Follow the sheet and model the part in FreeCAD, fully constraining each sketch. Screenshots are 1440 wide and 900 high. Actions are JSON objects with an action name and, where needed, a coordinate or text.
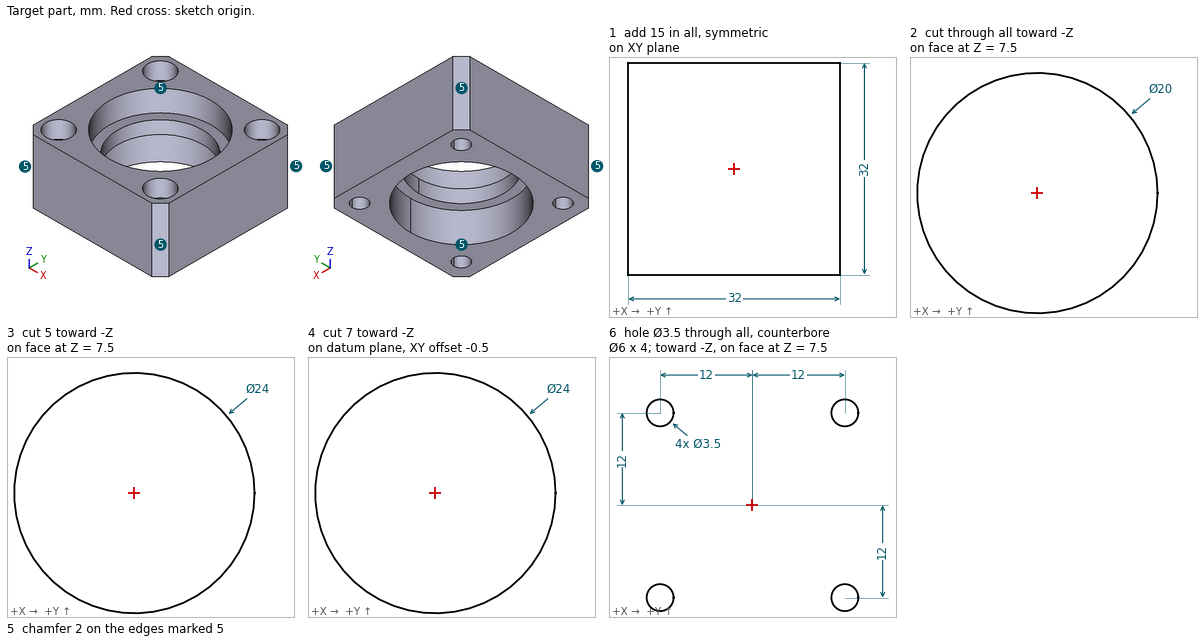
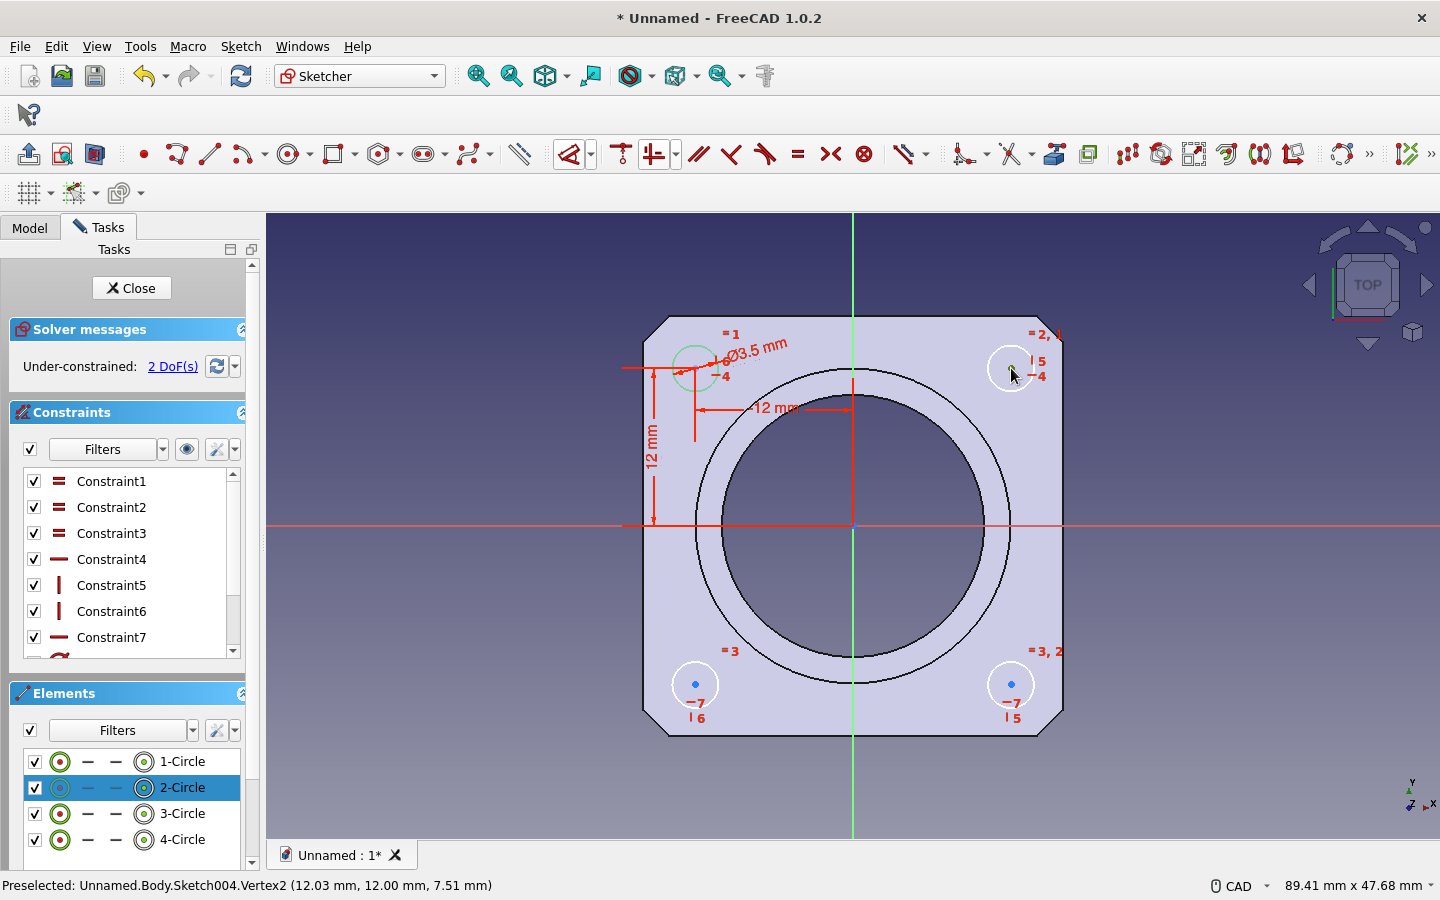
{"action": "left_click", "coordinate": [590, 154]}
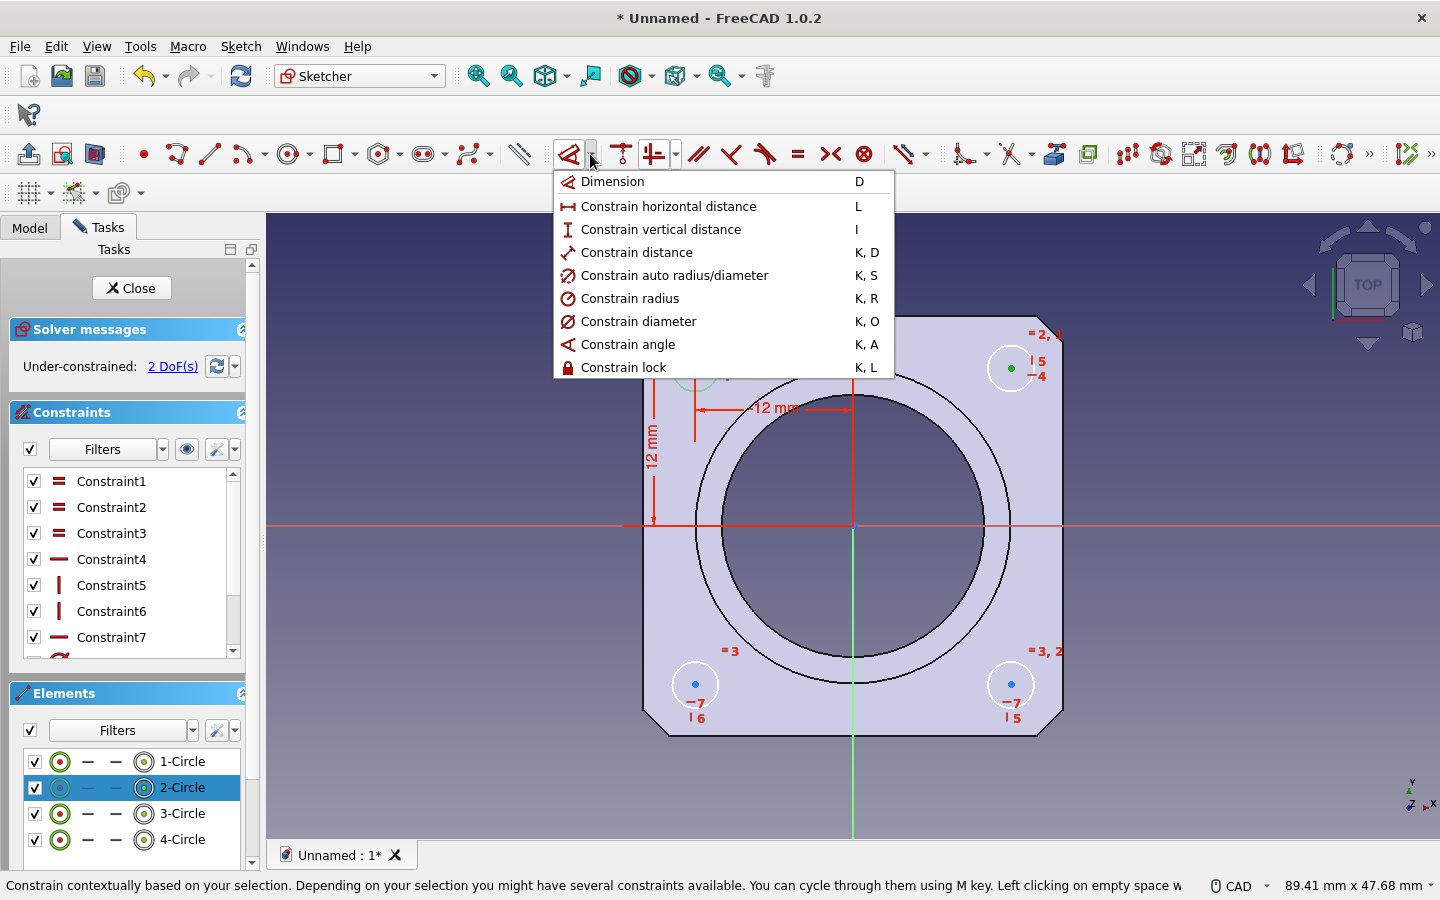
{"action": "left_click", "coordinate": [724, 206]}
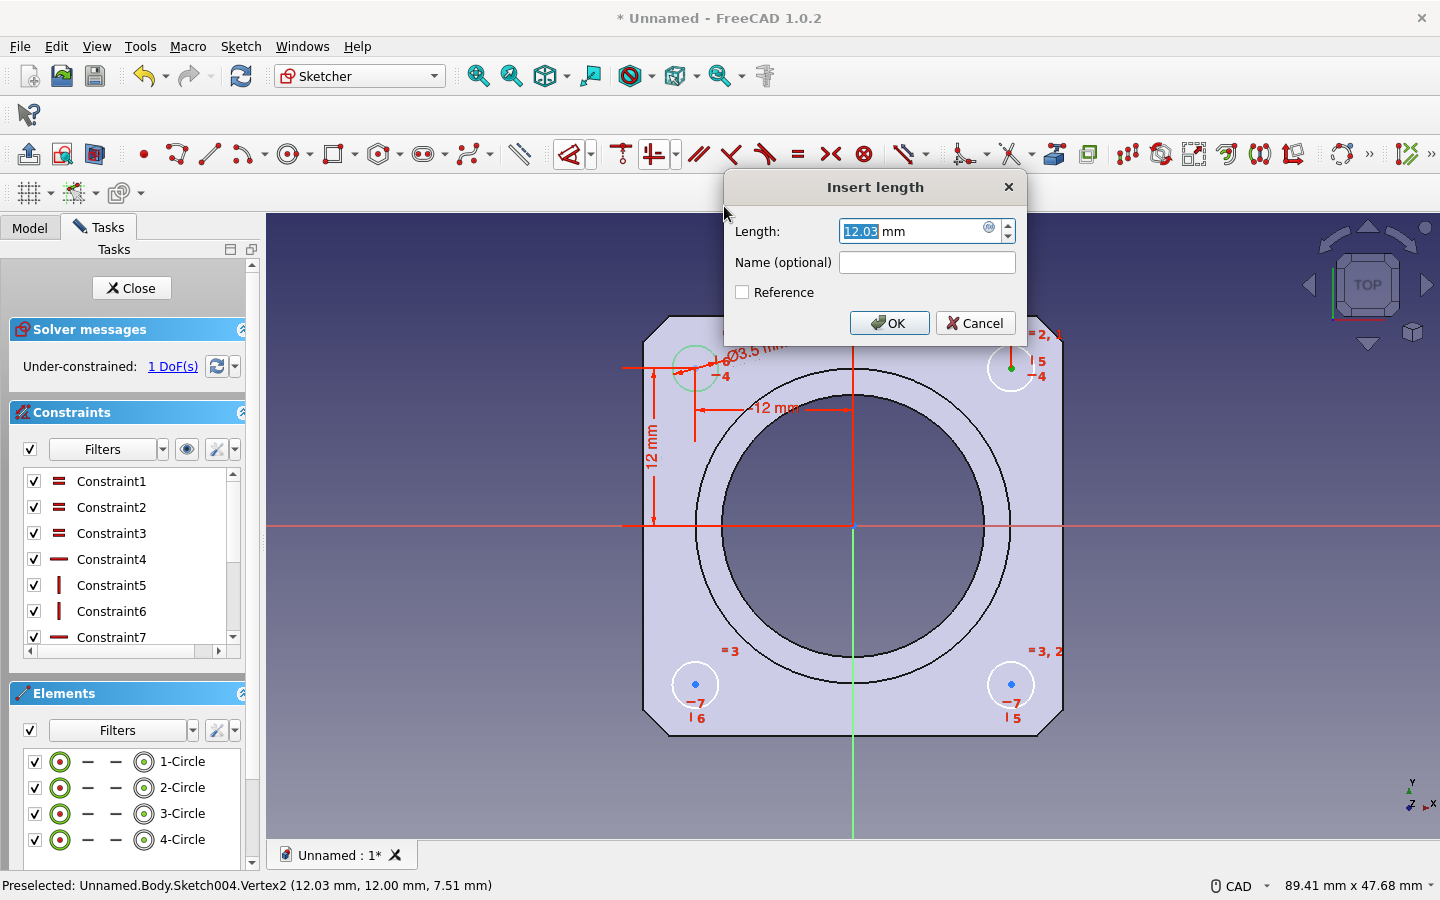
{"action": "type", "text": "12"}
{"action": "key", "text": "Return"}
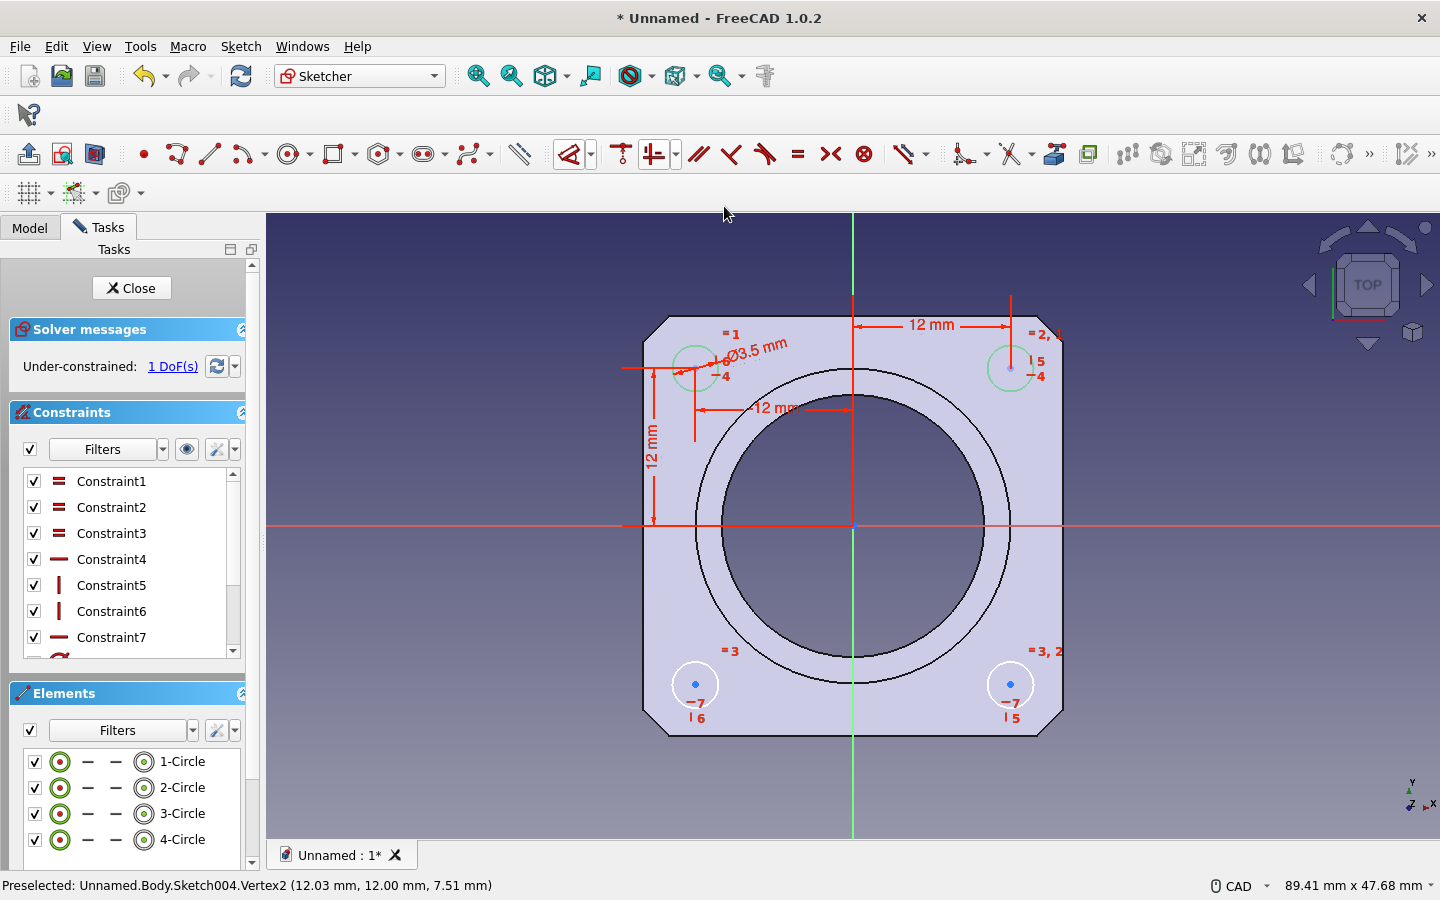
{"action": "left_click", "coordinate": [1011, 685]}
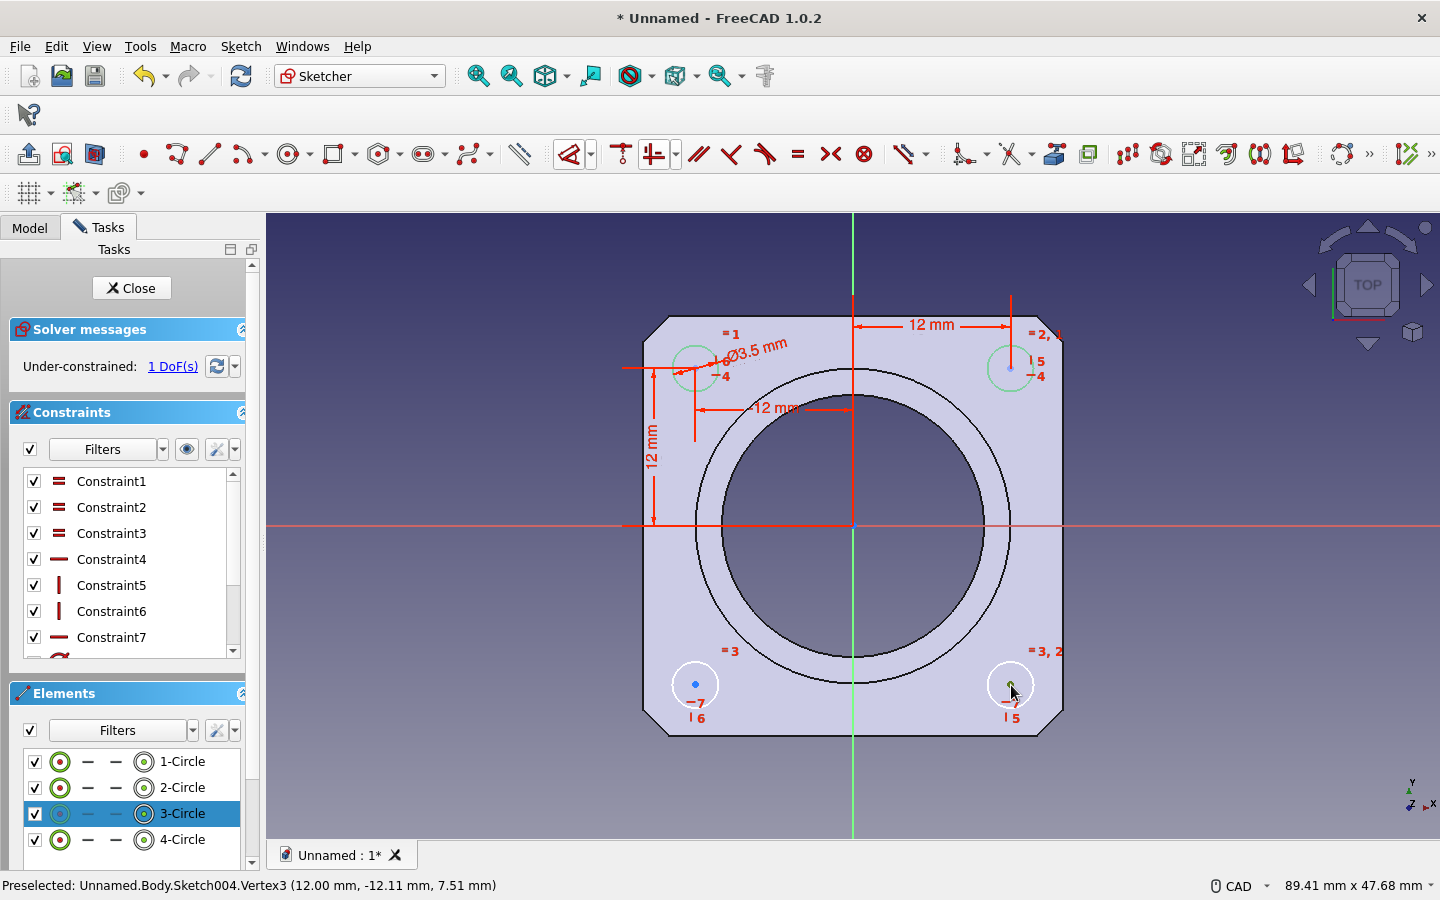
{"action": "key", "text": "i"}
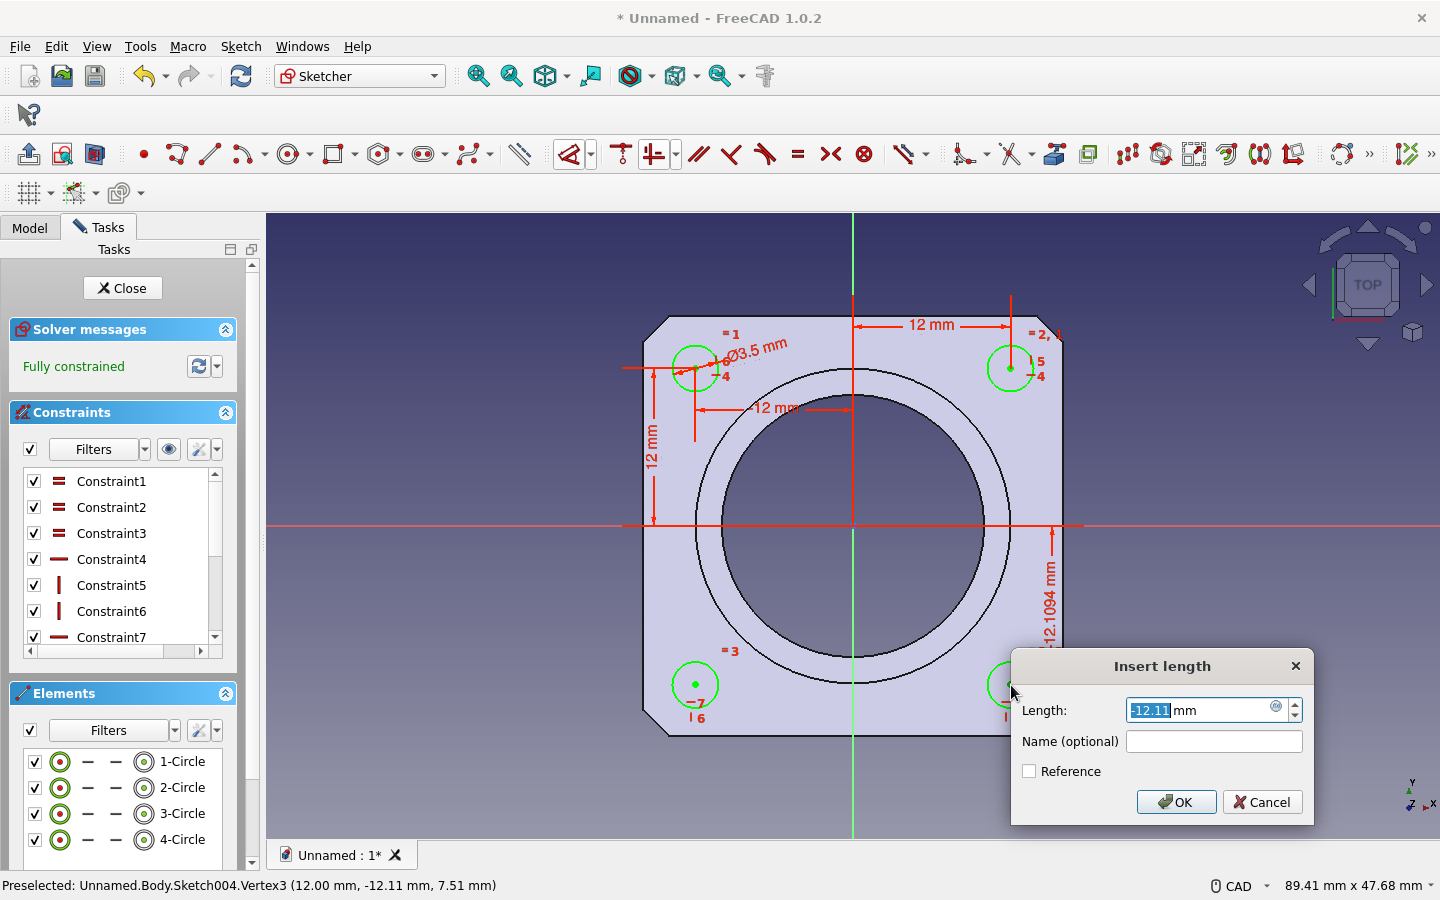
{"action": "type", "text": "-12"}
{"action": "key", "text": "Return"}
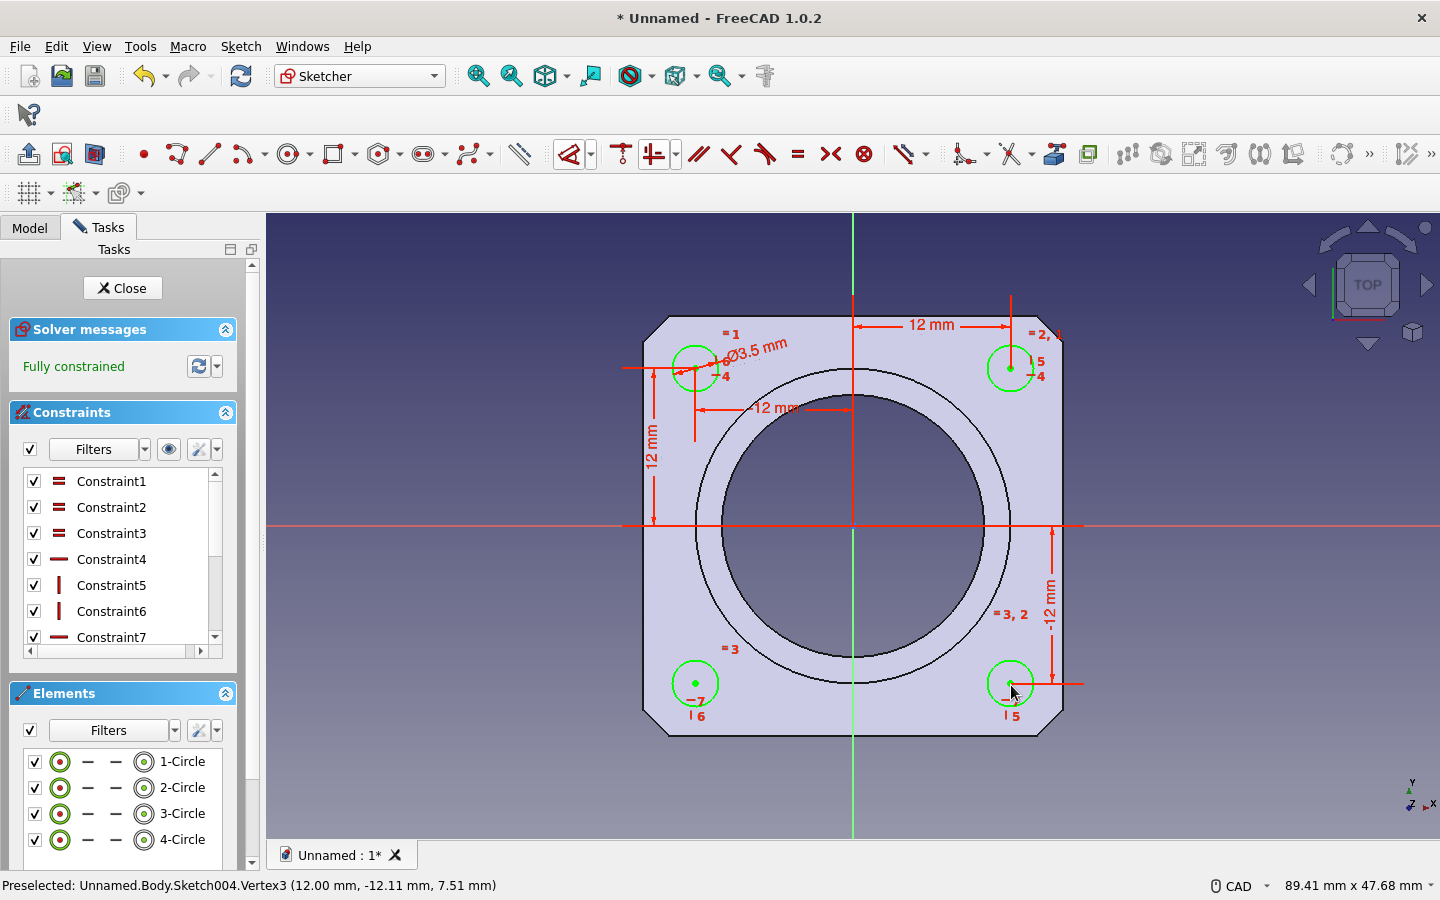
{"action": "left_click", "coordinate": [123, 288]}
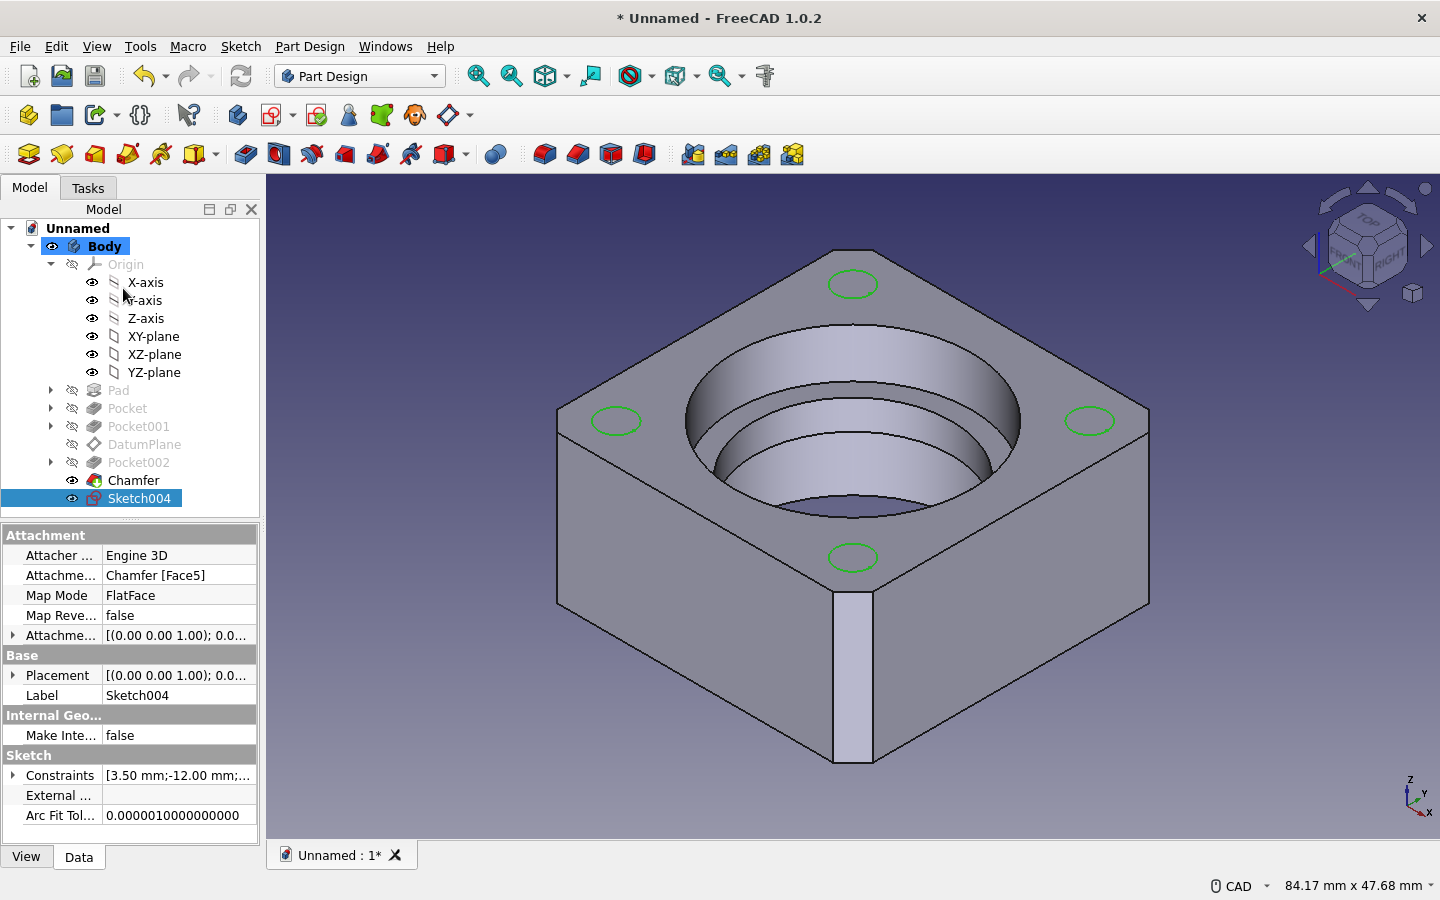
{"action": "left_click", "coordinate": [279, 154]}